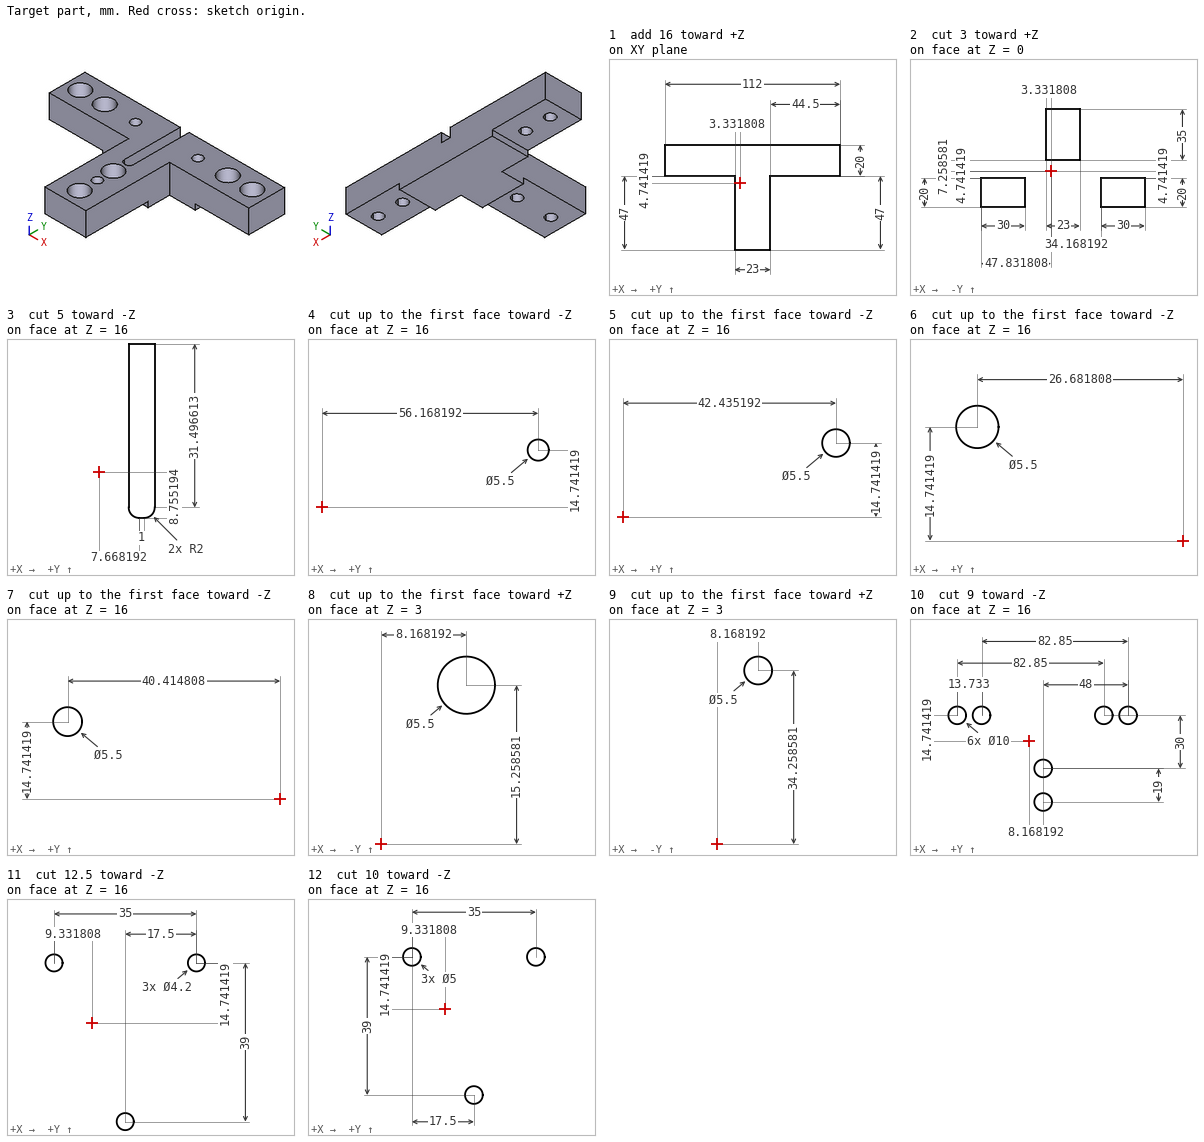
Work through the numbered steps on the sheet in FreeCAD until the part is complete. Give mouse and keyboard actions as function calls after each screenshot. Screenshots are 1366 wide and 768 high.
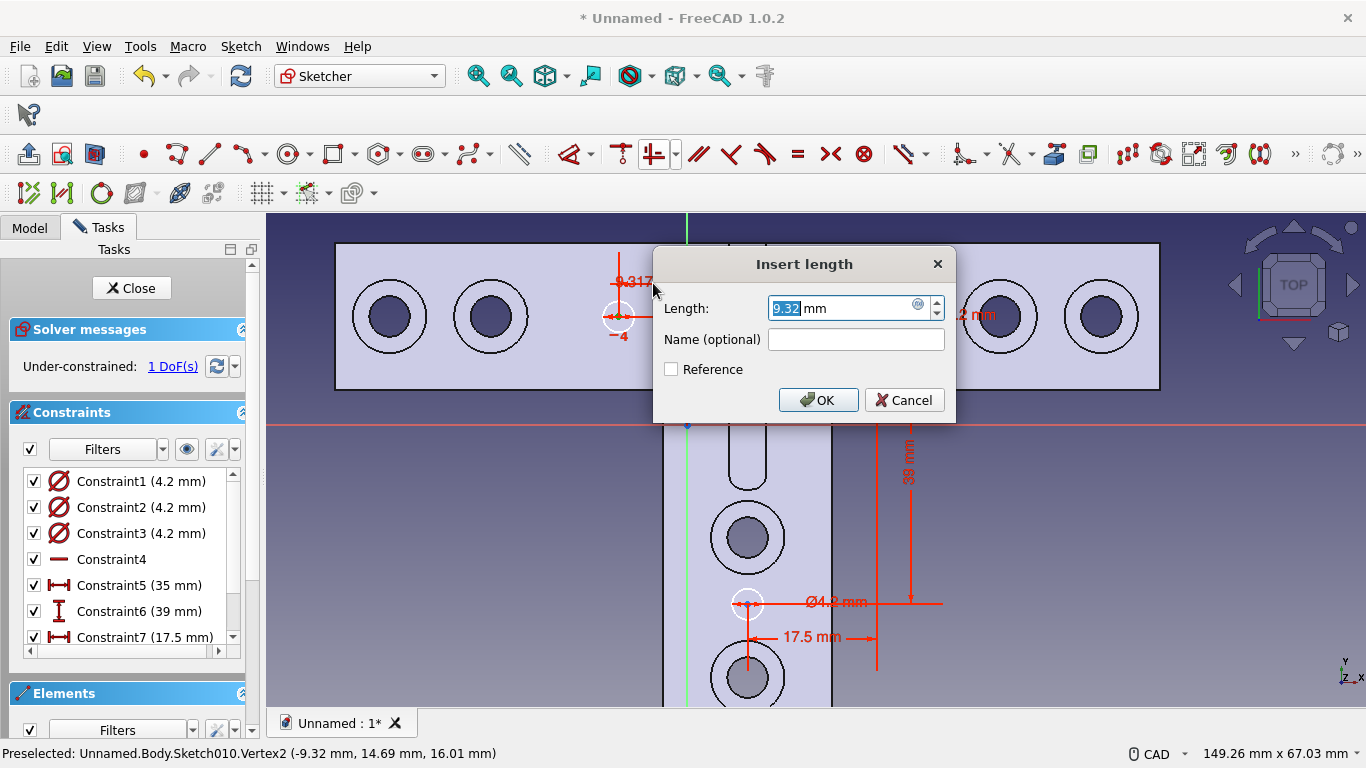
text(9.331808)
key(Return)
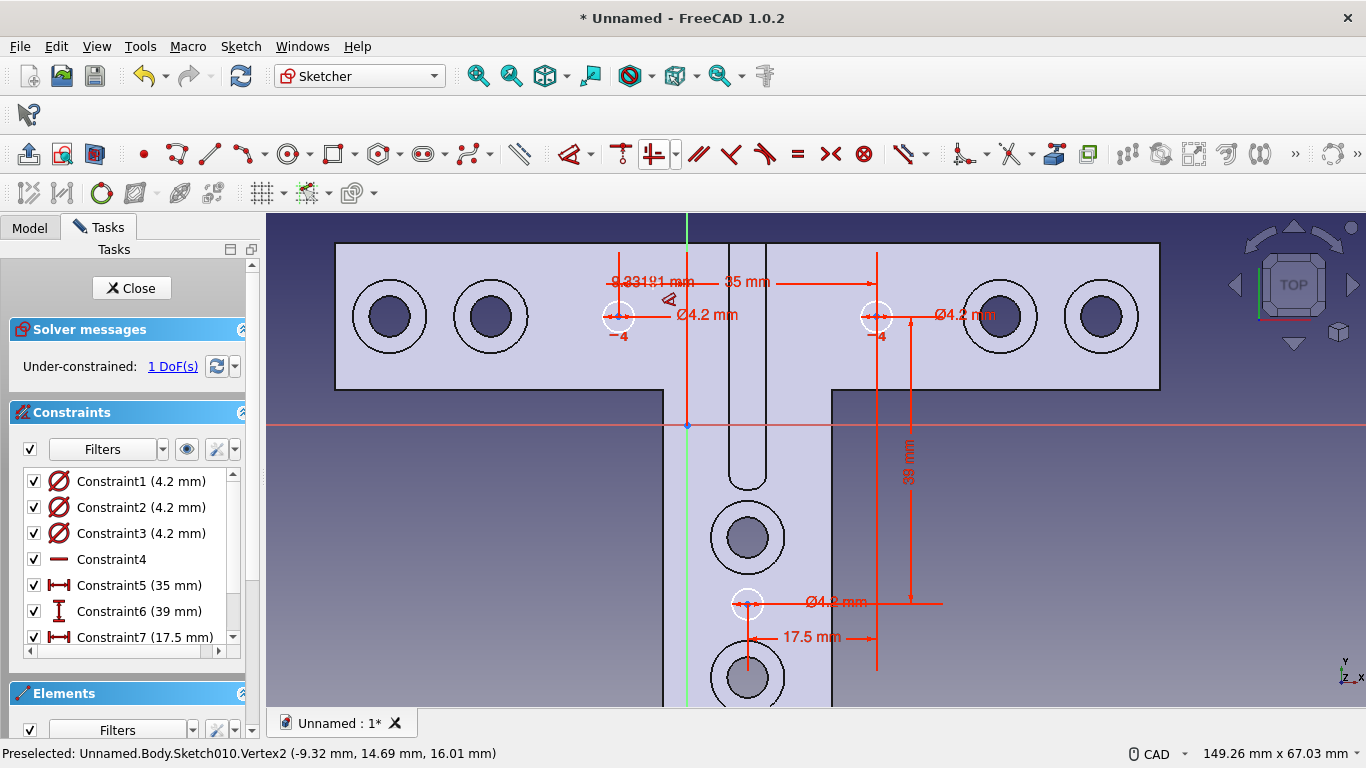
click(877, 317)
click(911, 371)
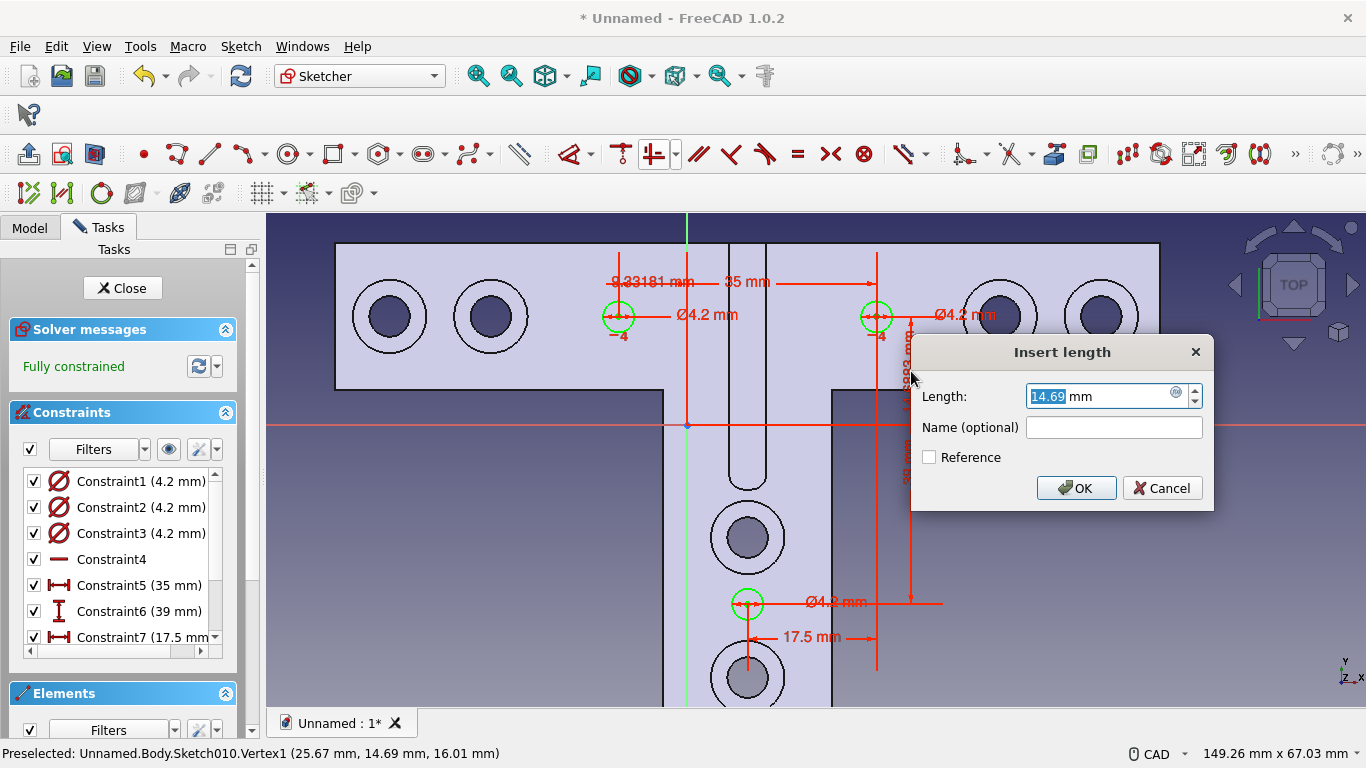
text(14.741419)
key(Return)
key(Escape)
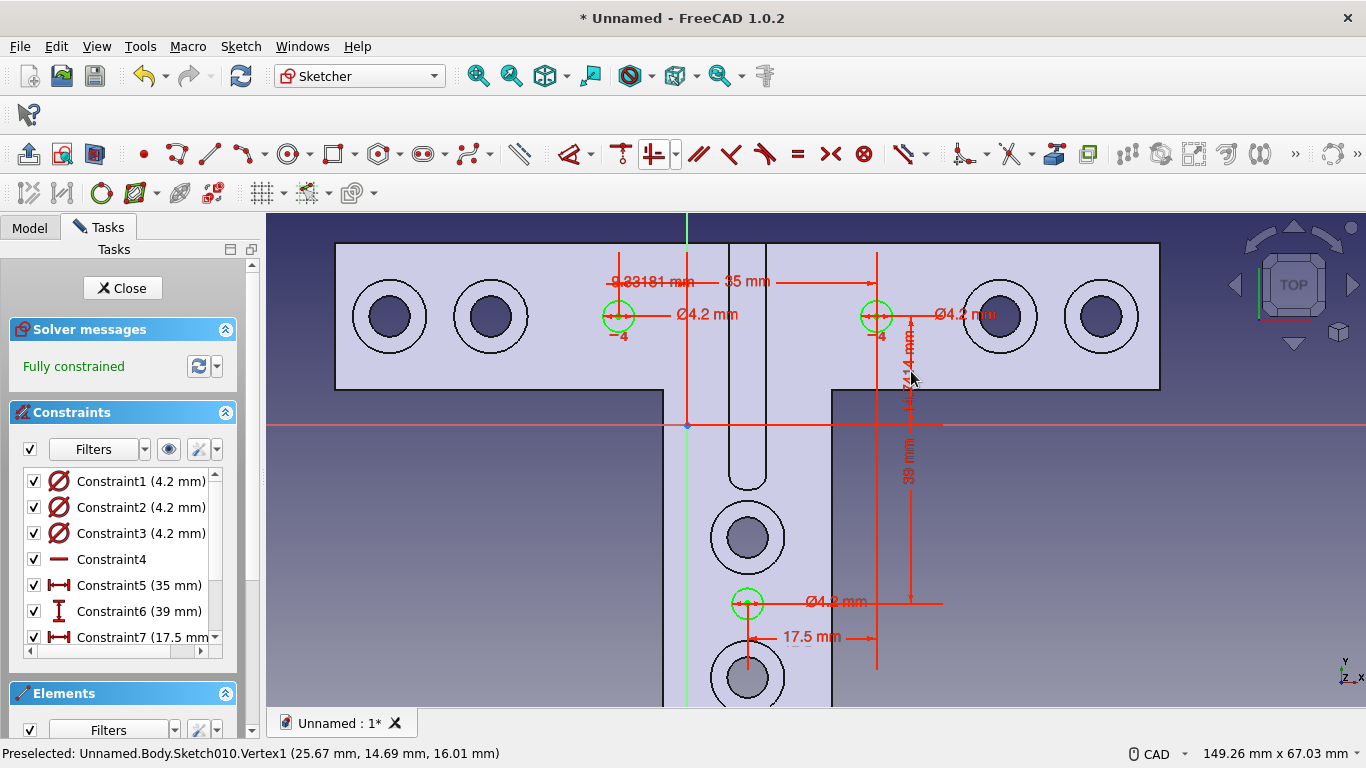
click(123, 288)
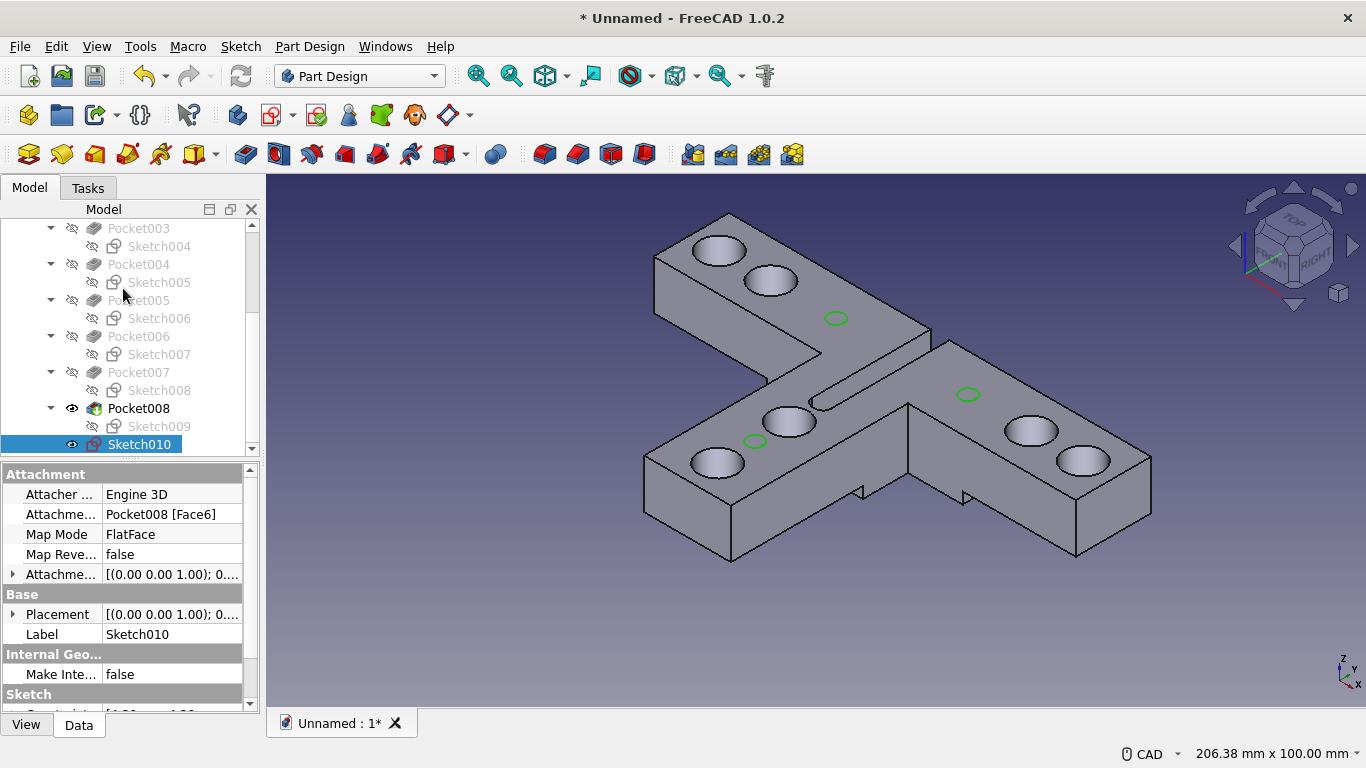
click(246, 154)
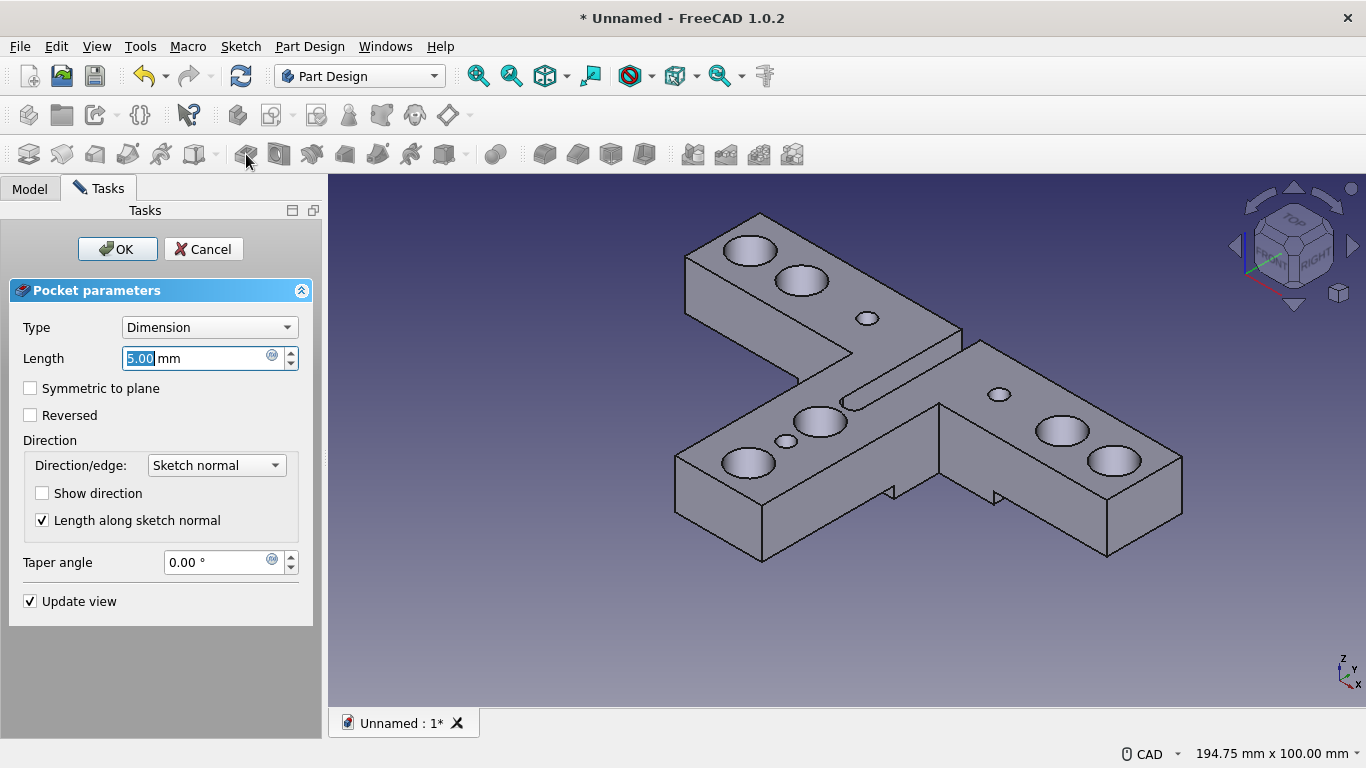
text(12.5)
key(Tab)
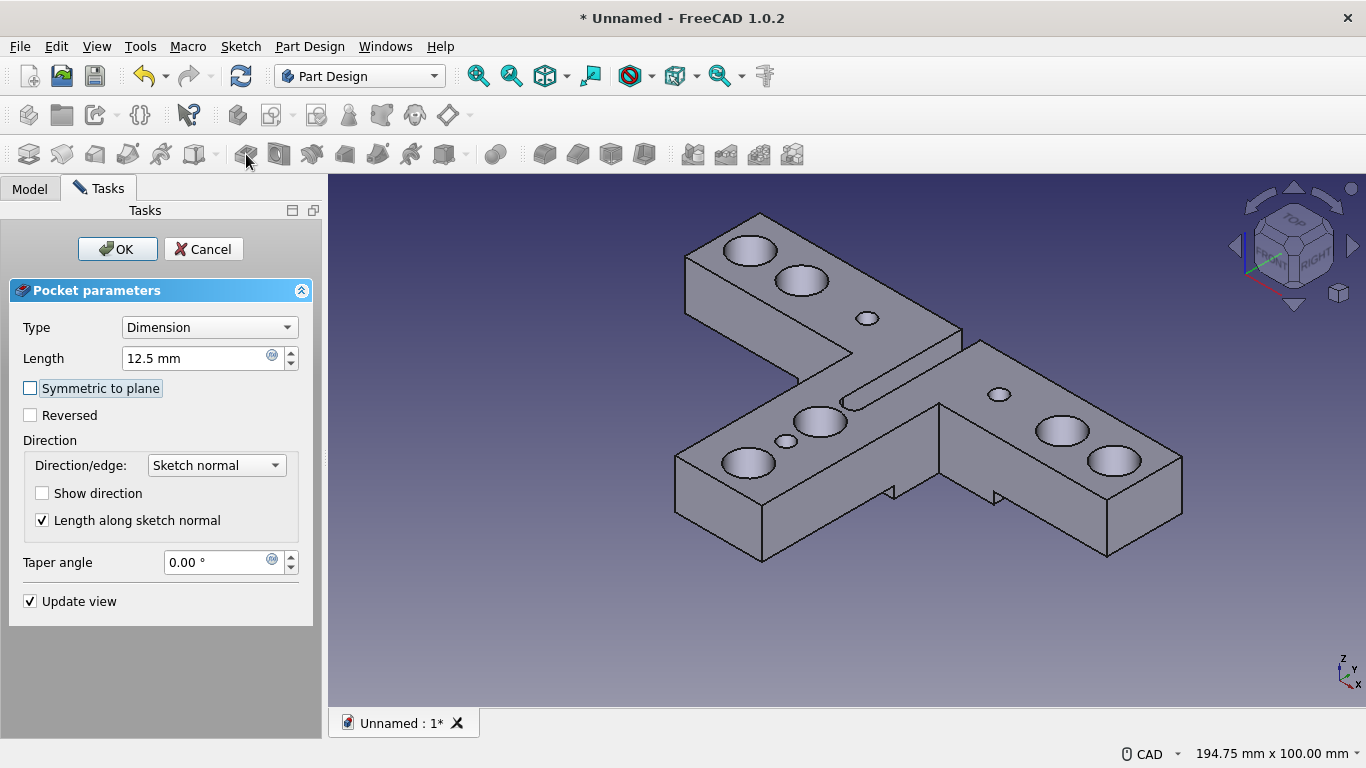
click(118, 249)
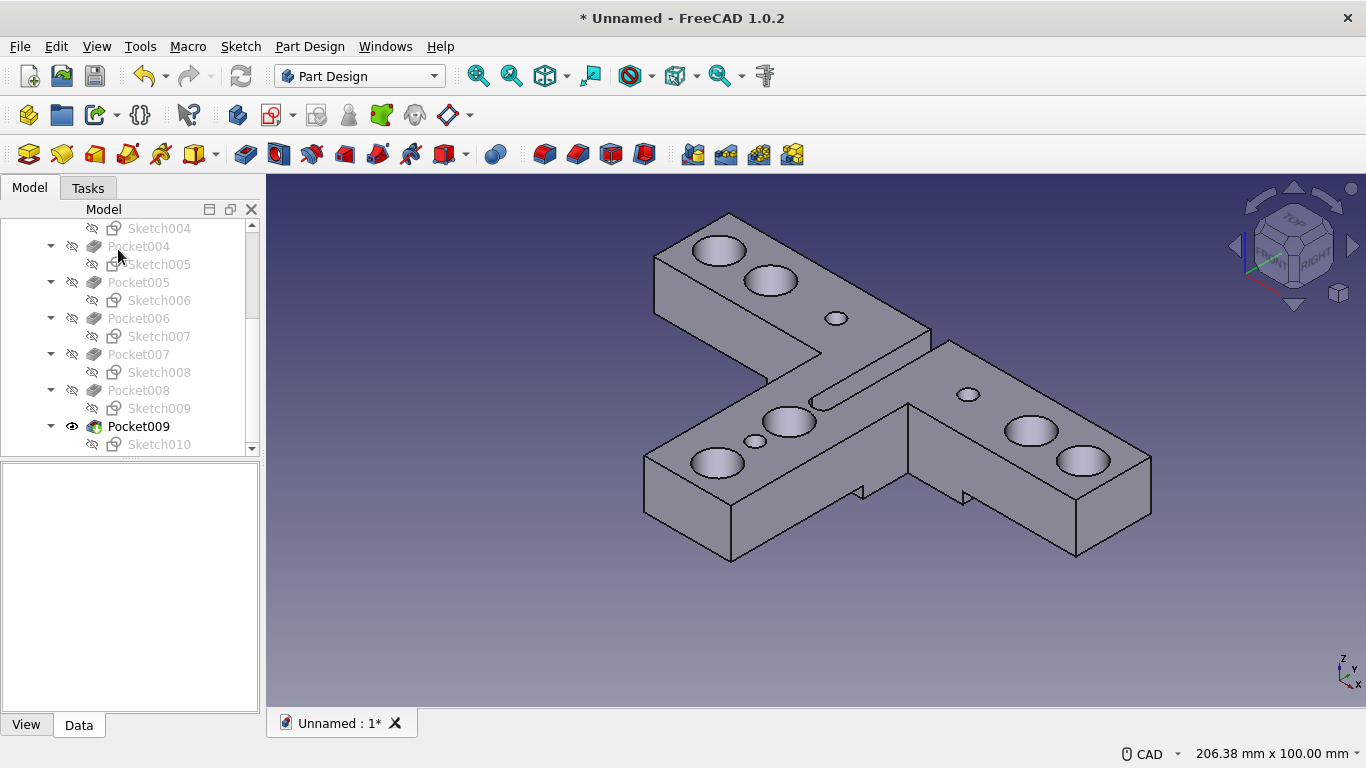
click(862, 309)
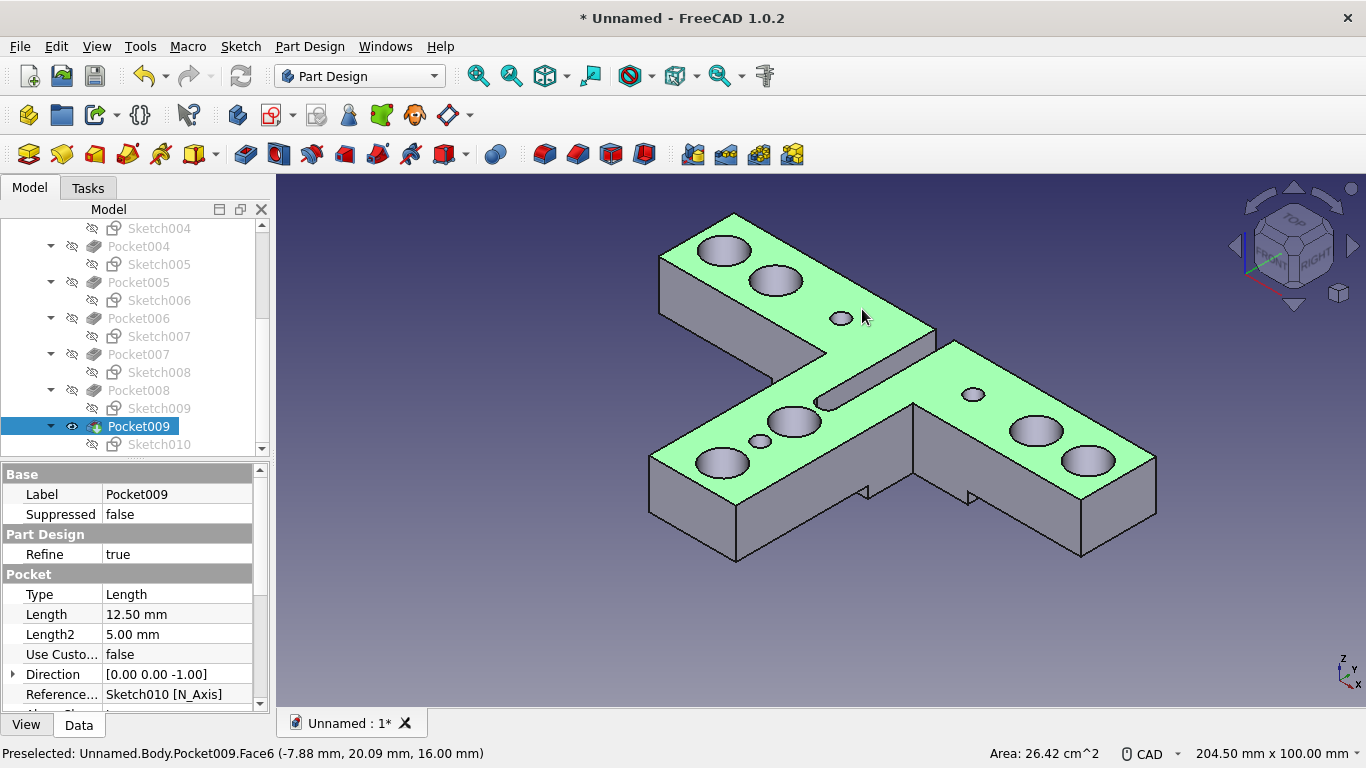
click(270, 116)